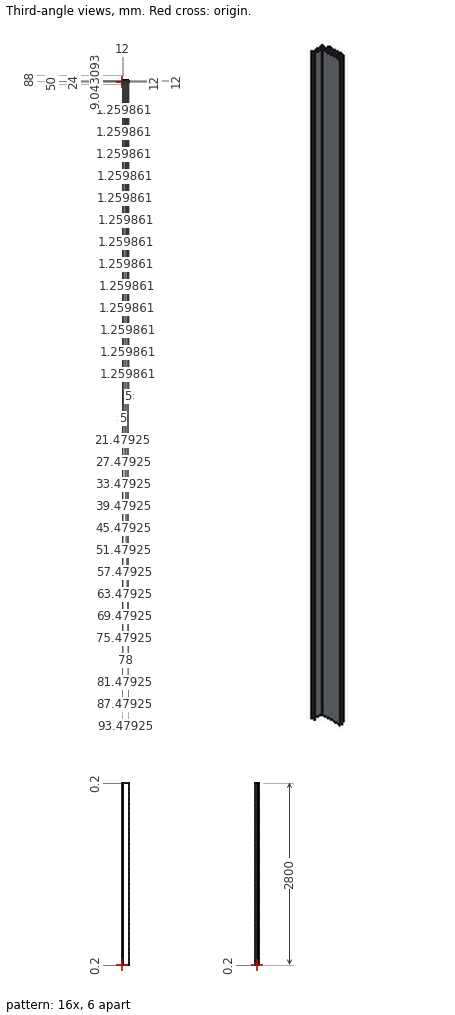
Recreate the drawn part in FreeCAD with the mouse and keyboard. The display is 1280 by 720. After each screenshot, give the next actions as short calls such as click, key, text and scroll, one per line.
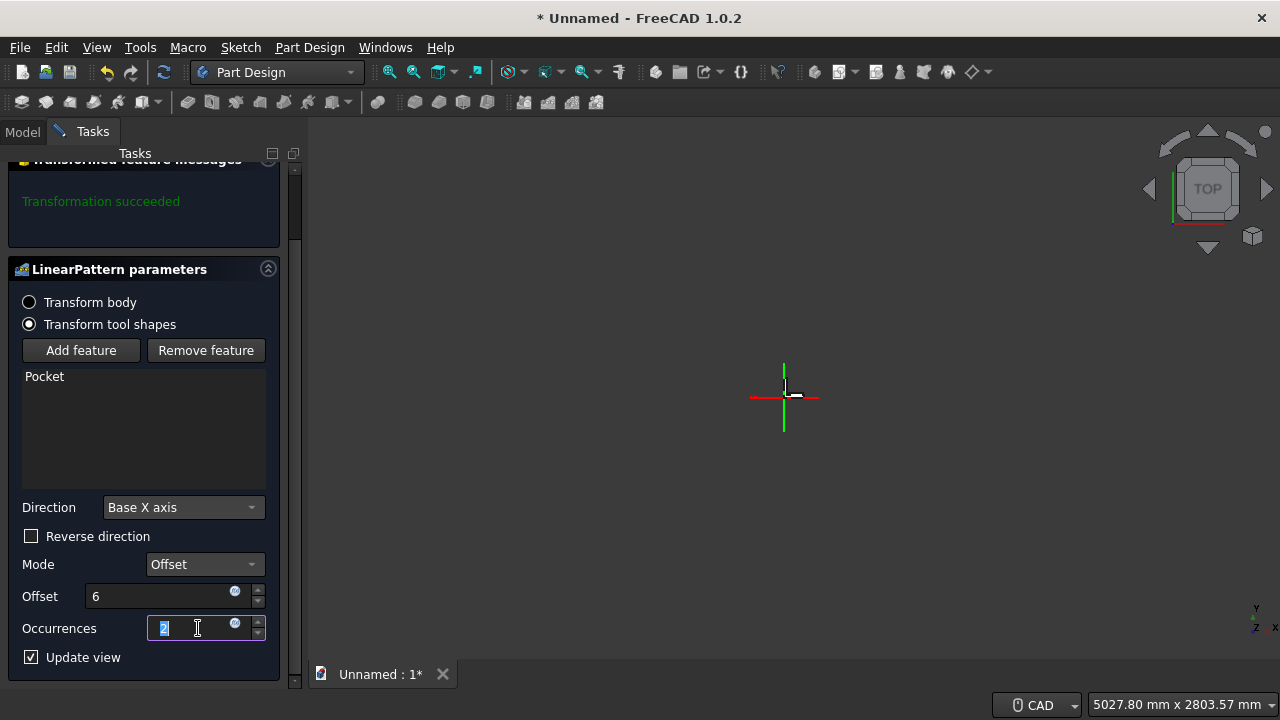
text(16)
key(Tab)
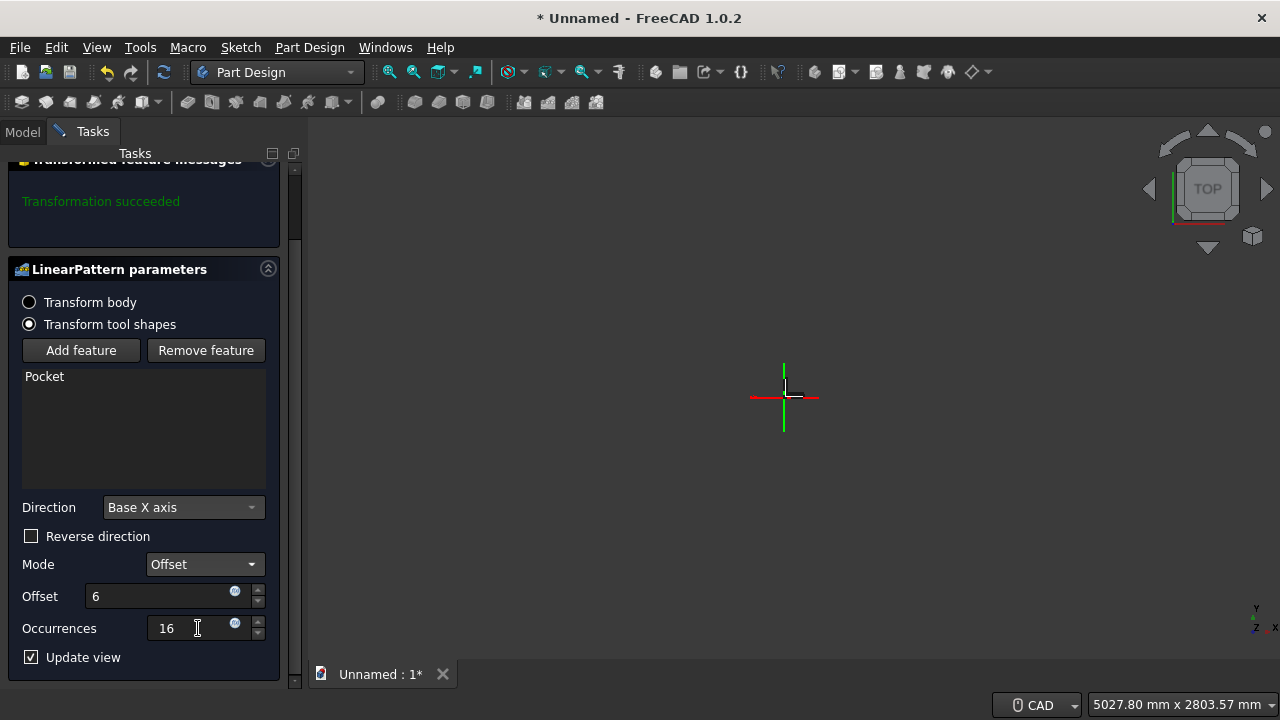
scroll(295, 426, up, 3)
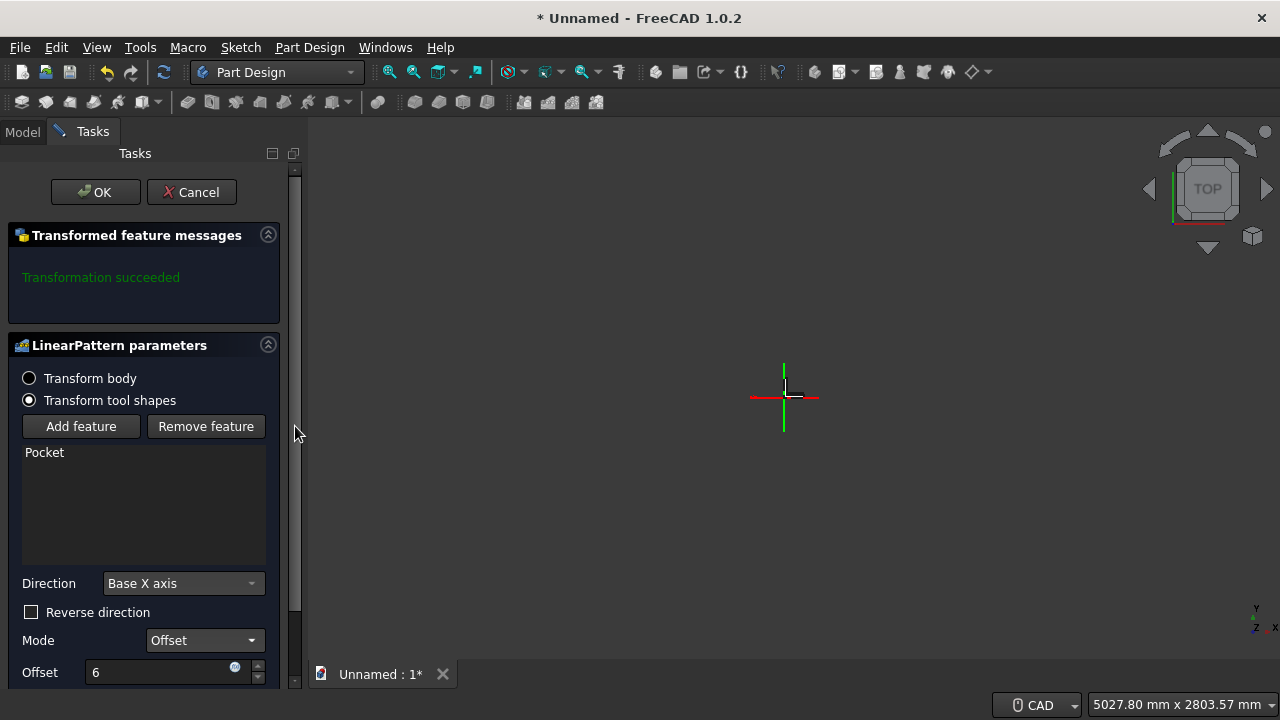
click(96, 192)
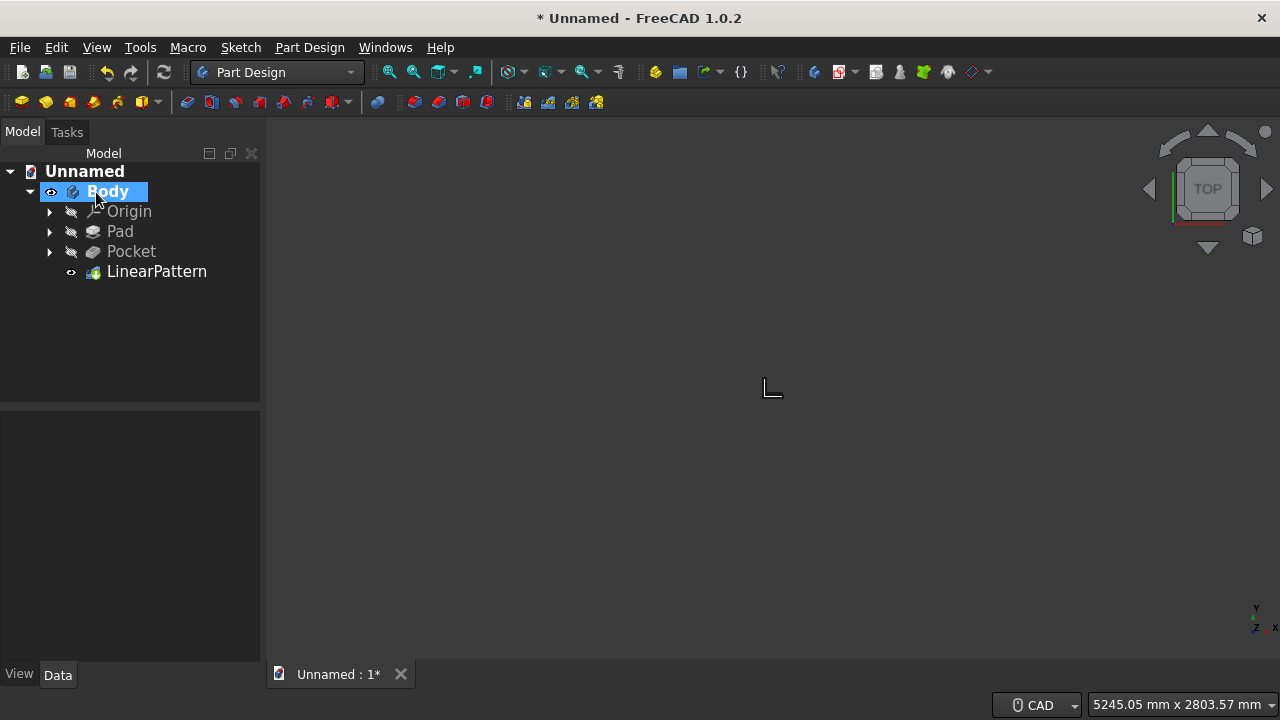
click(390, 72)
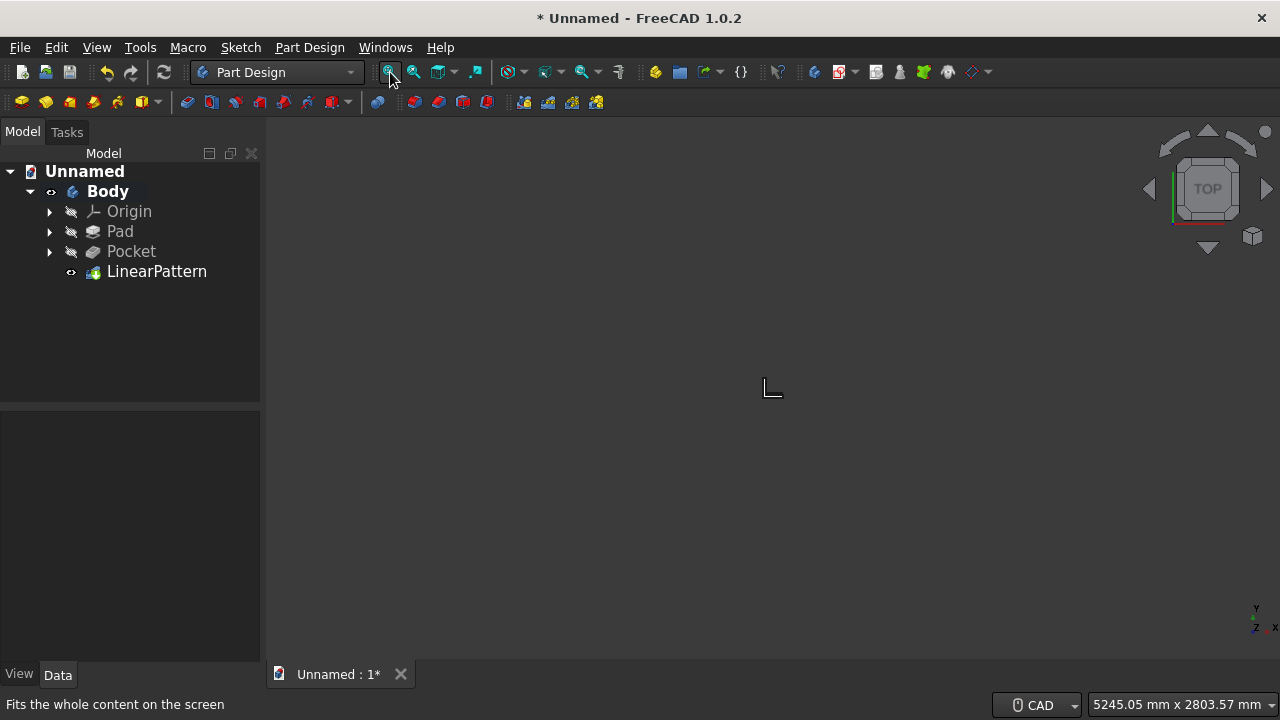
click(50, 212)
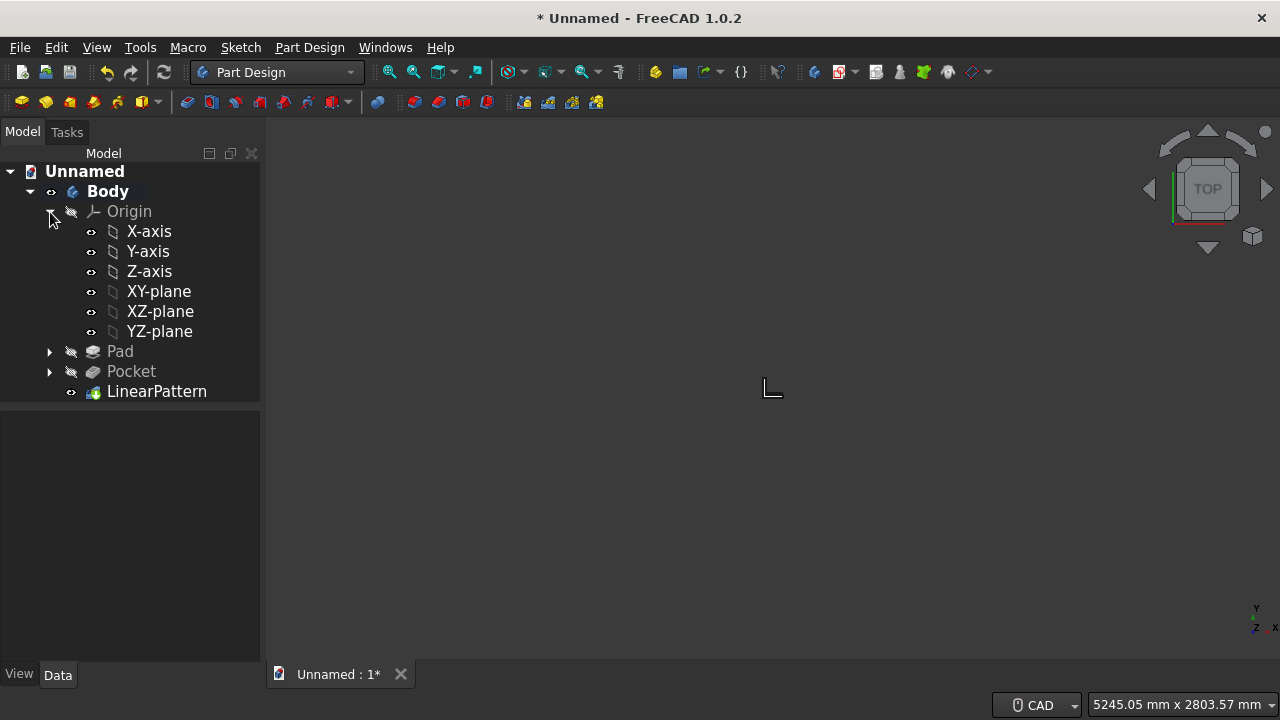
click(136, 292)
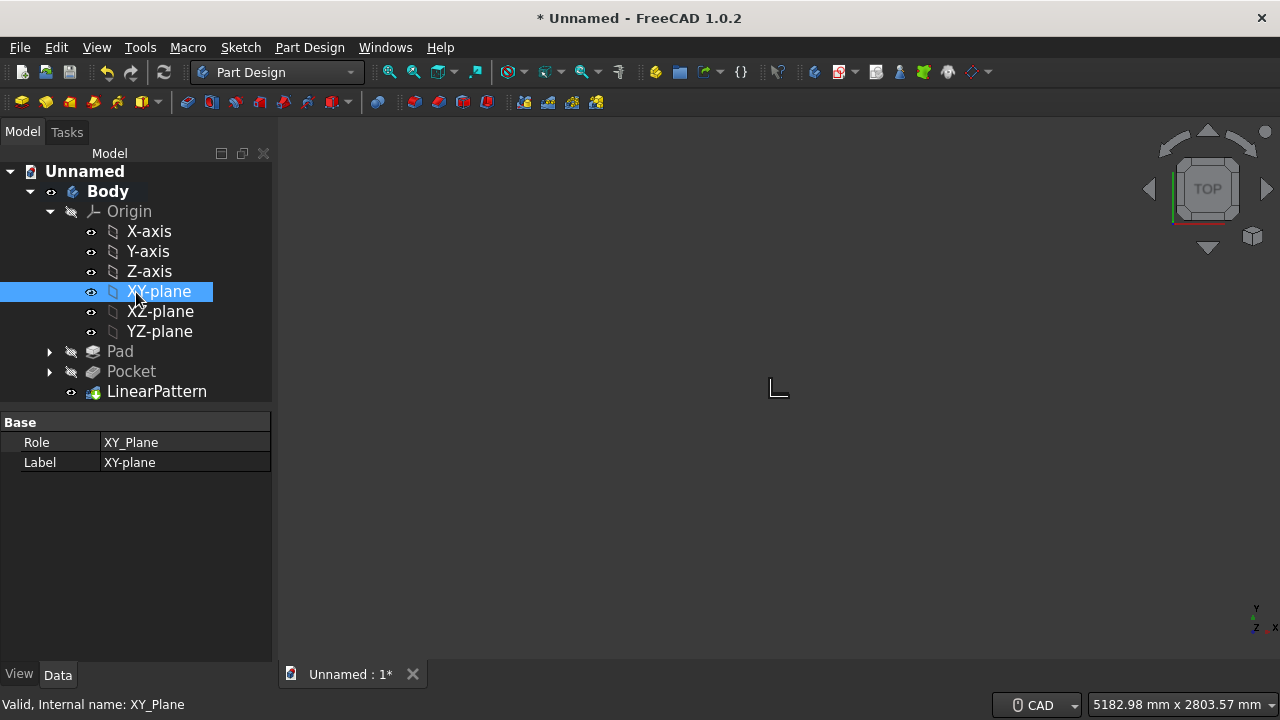
click(972, 72)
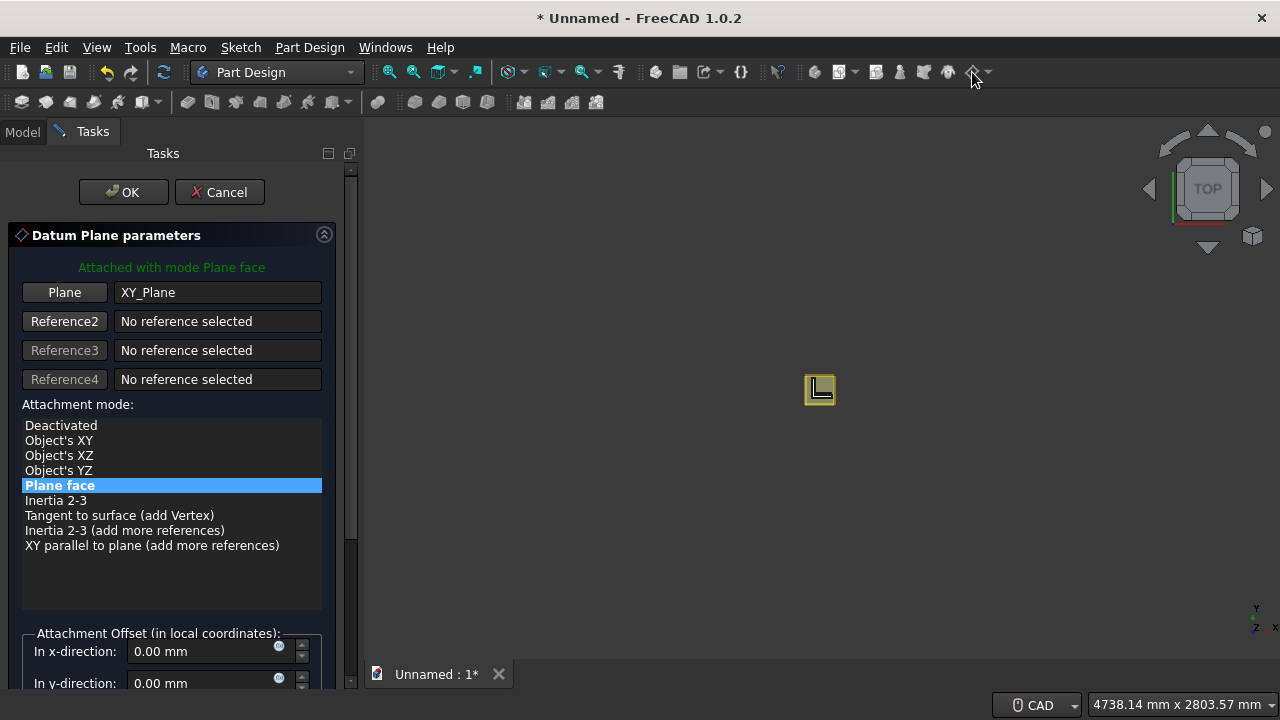
scroll(351, 426, down, 2)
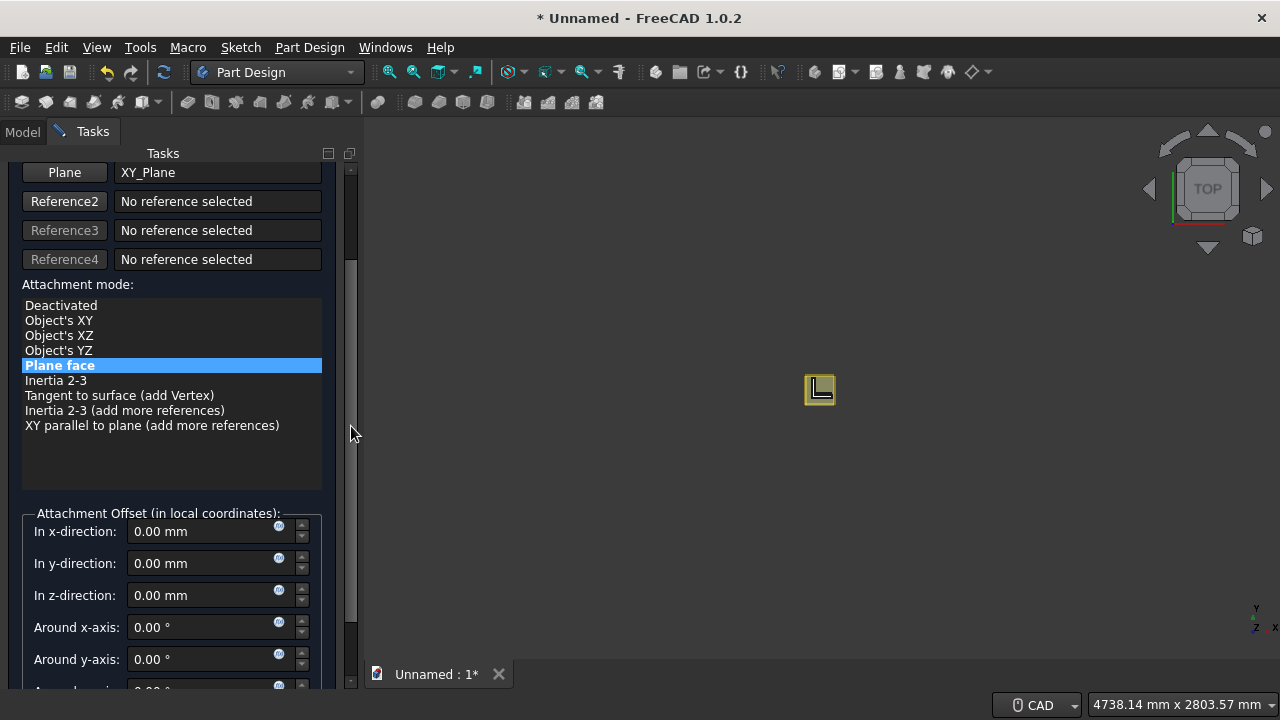
triple_click(210, 595)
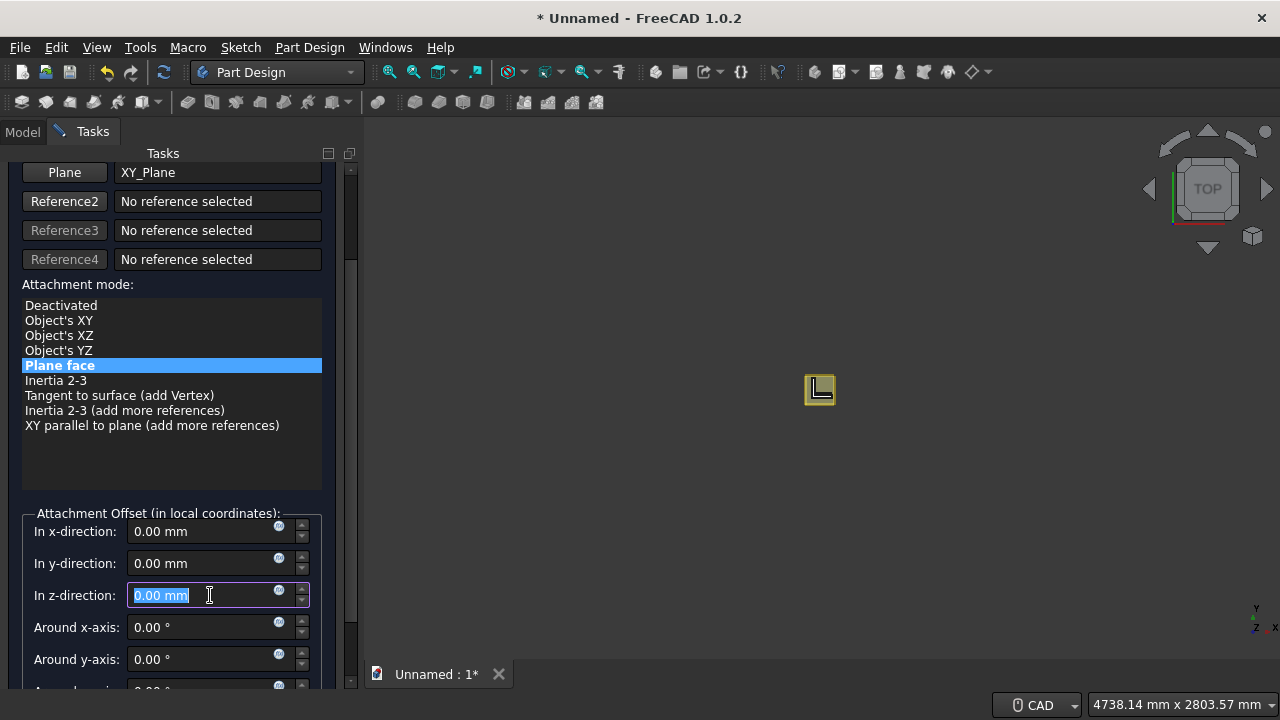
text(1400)
key(Tab)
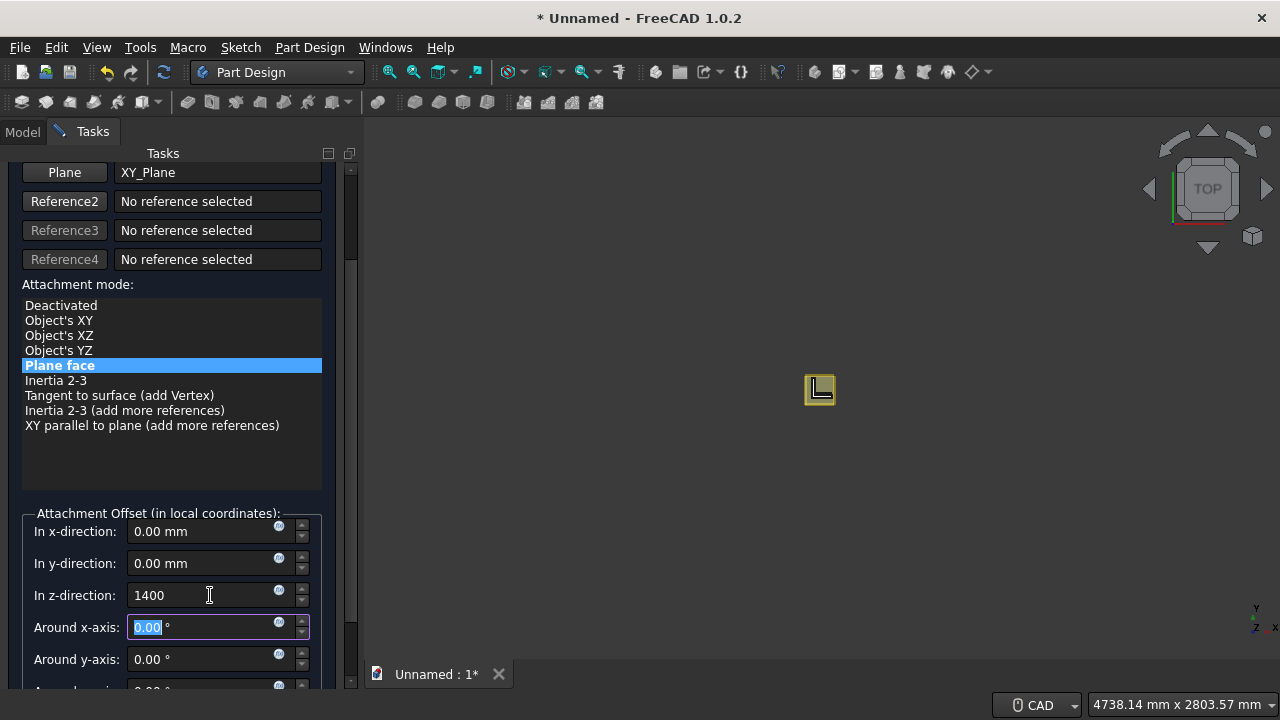
scroll(351, 426, up, 3)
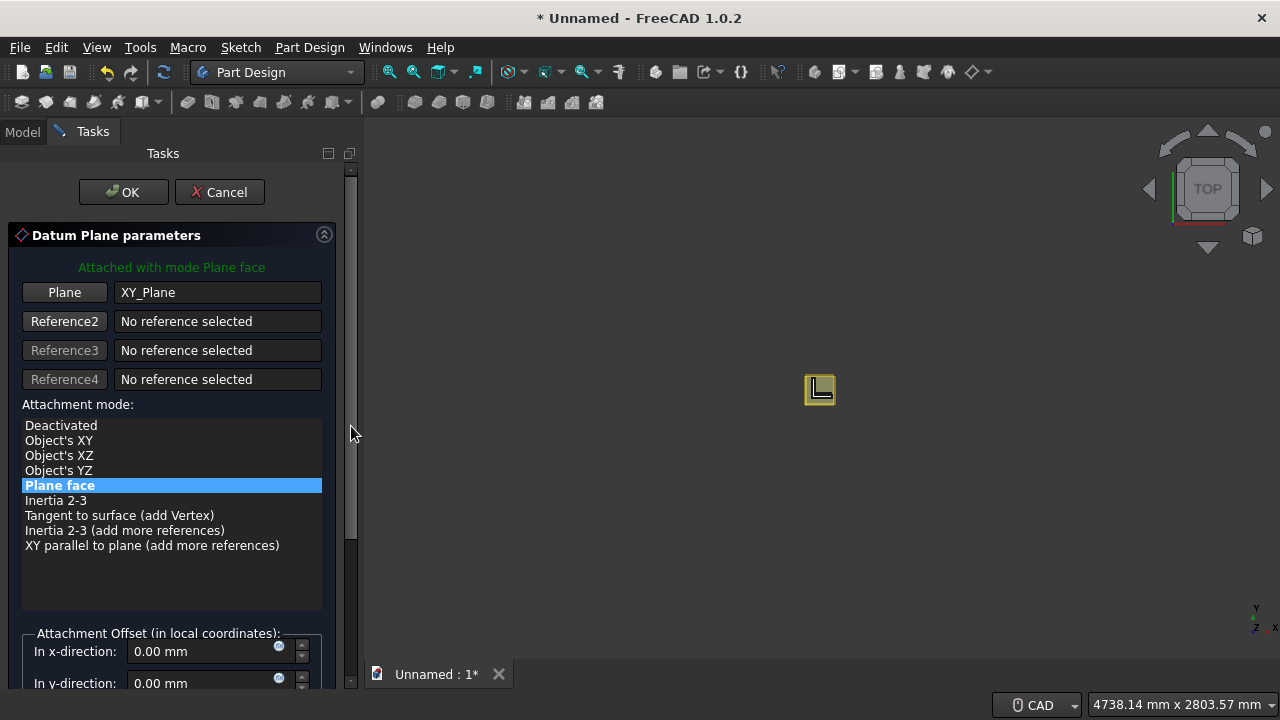
click(124, 192)